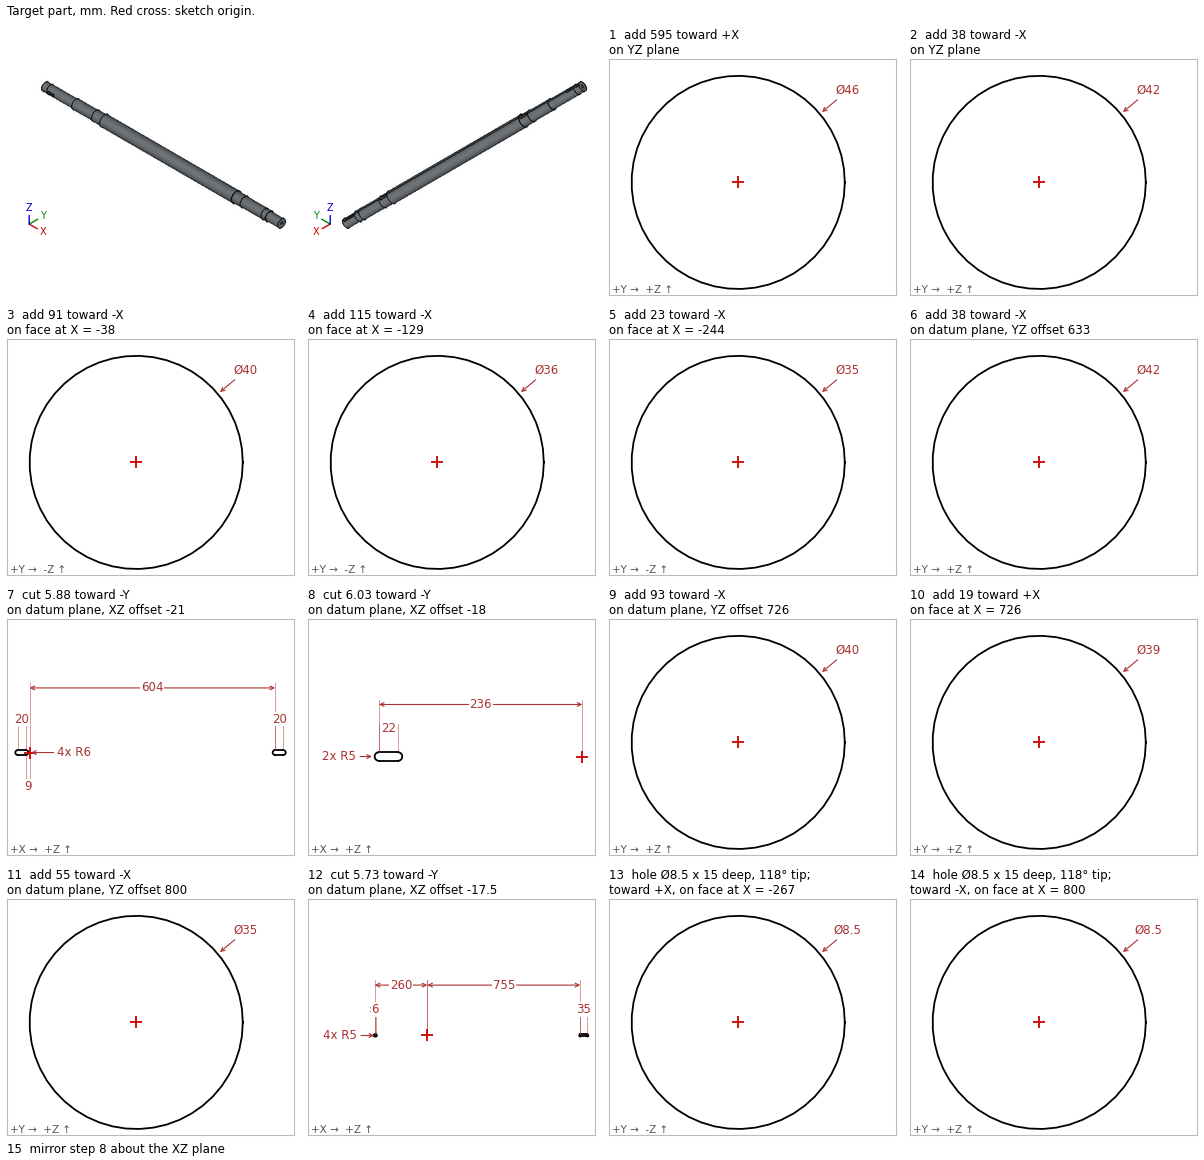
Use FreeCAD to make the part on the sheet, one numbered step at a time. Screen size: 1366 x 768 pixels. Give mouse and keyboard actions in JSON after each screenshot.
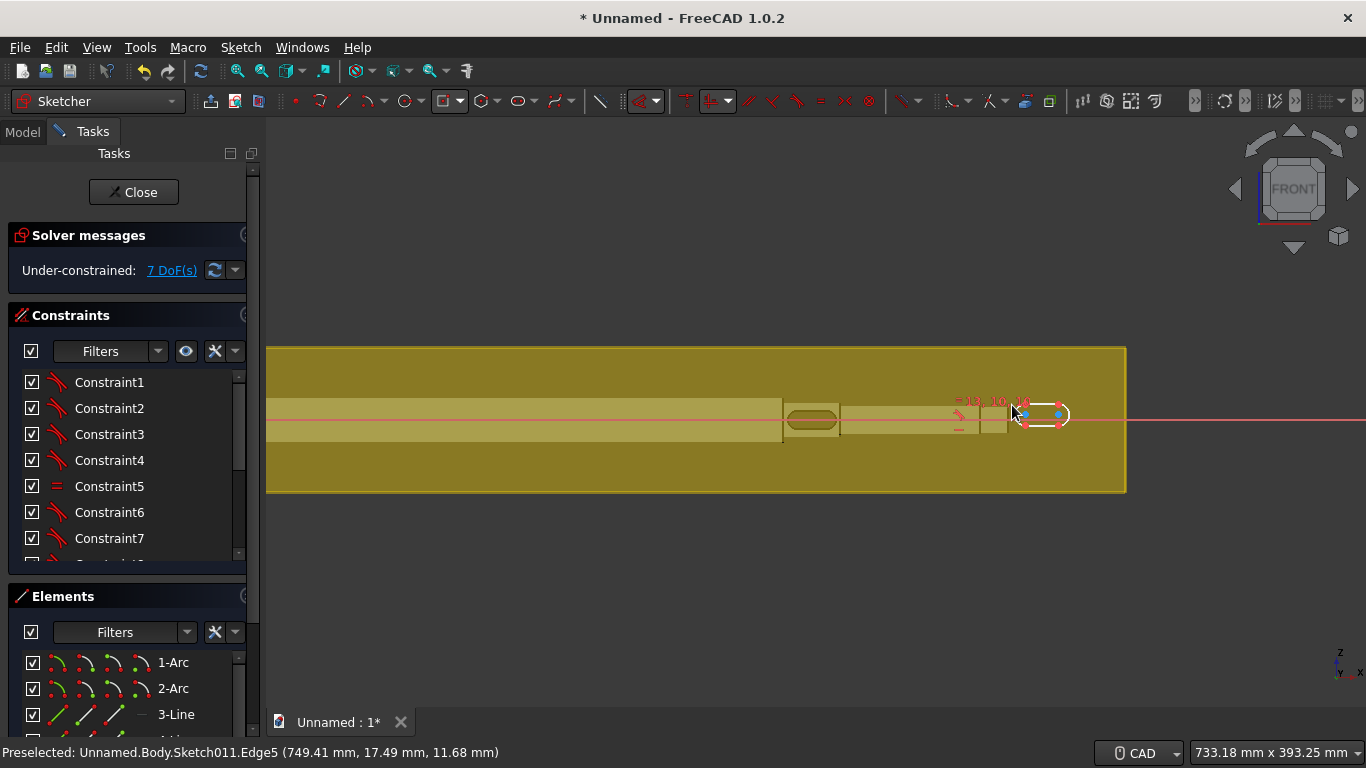
{"action": "scroll", "coordinate": [1015, 407], "scroll_direction": "down", "scroll_amount": 5}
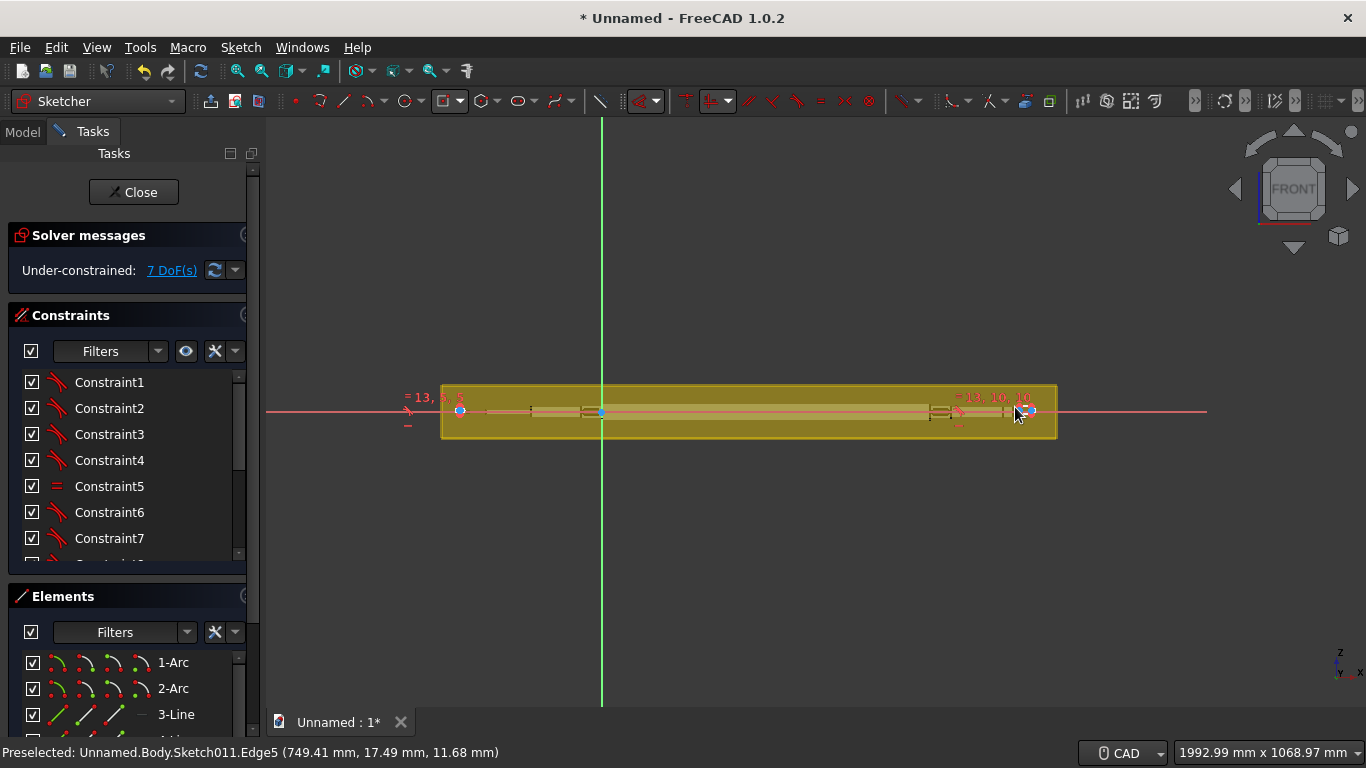
{"action": "scroll", "coordinate": [460, 411], "scroll_direction": "up", "scroll_amount": 14}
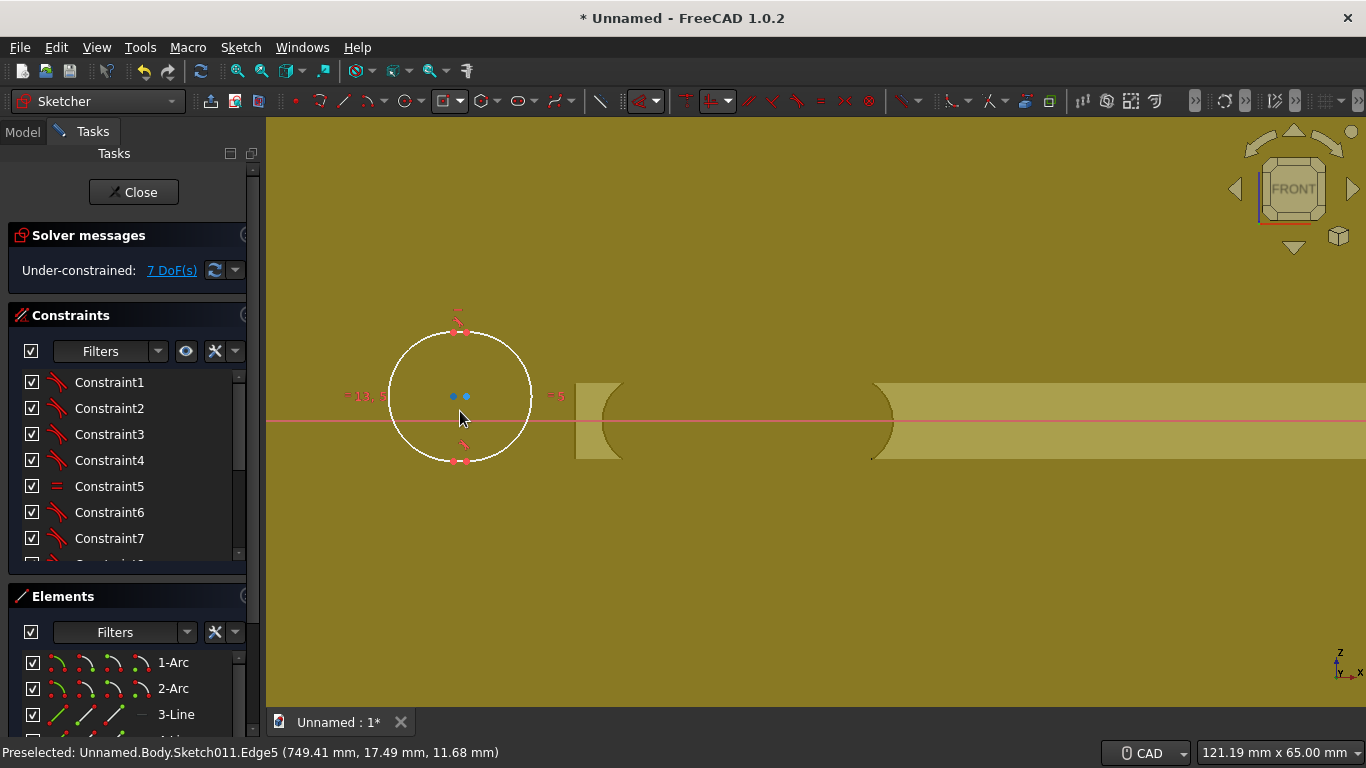
{"action": "left_click", "coordinate": [453, 397]}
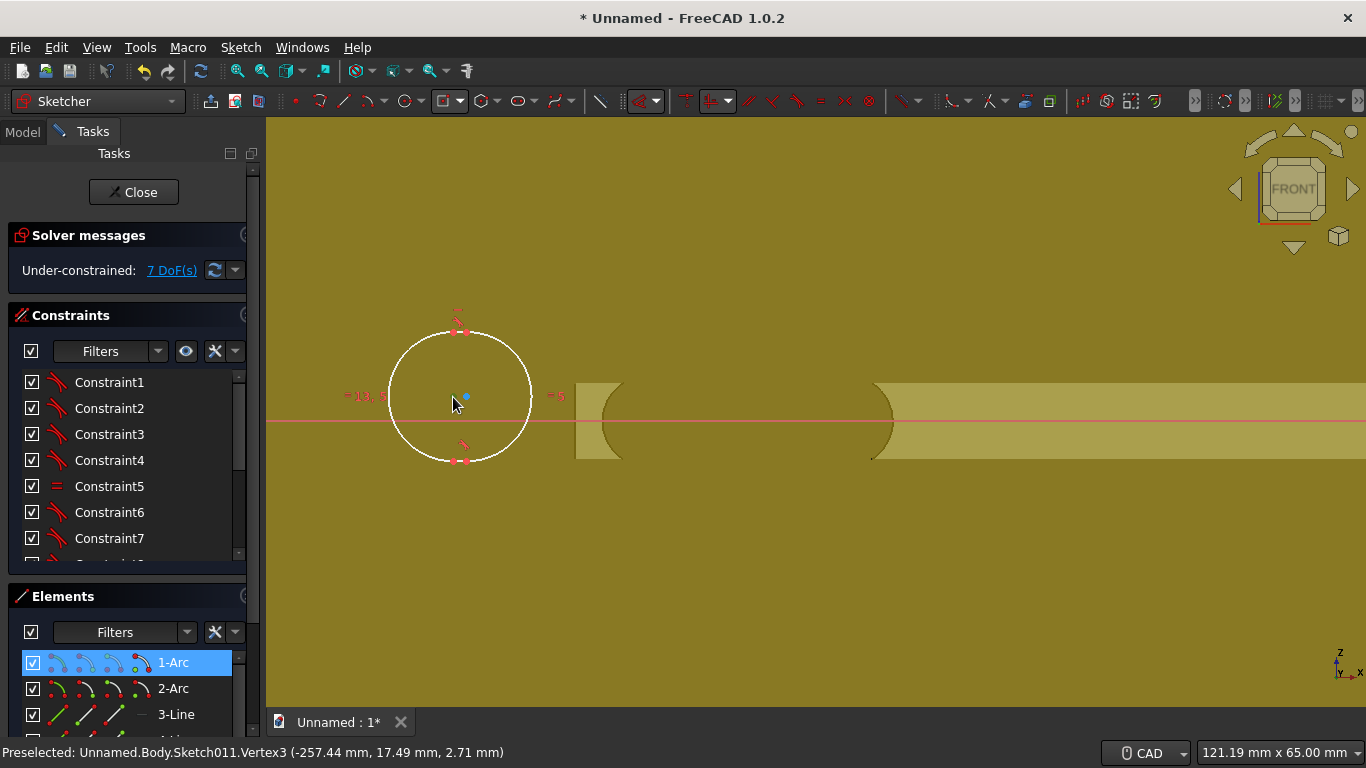
{"action": "left_click", "coordinate": [359, 421]}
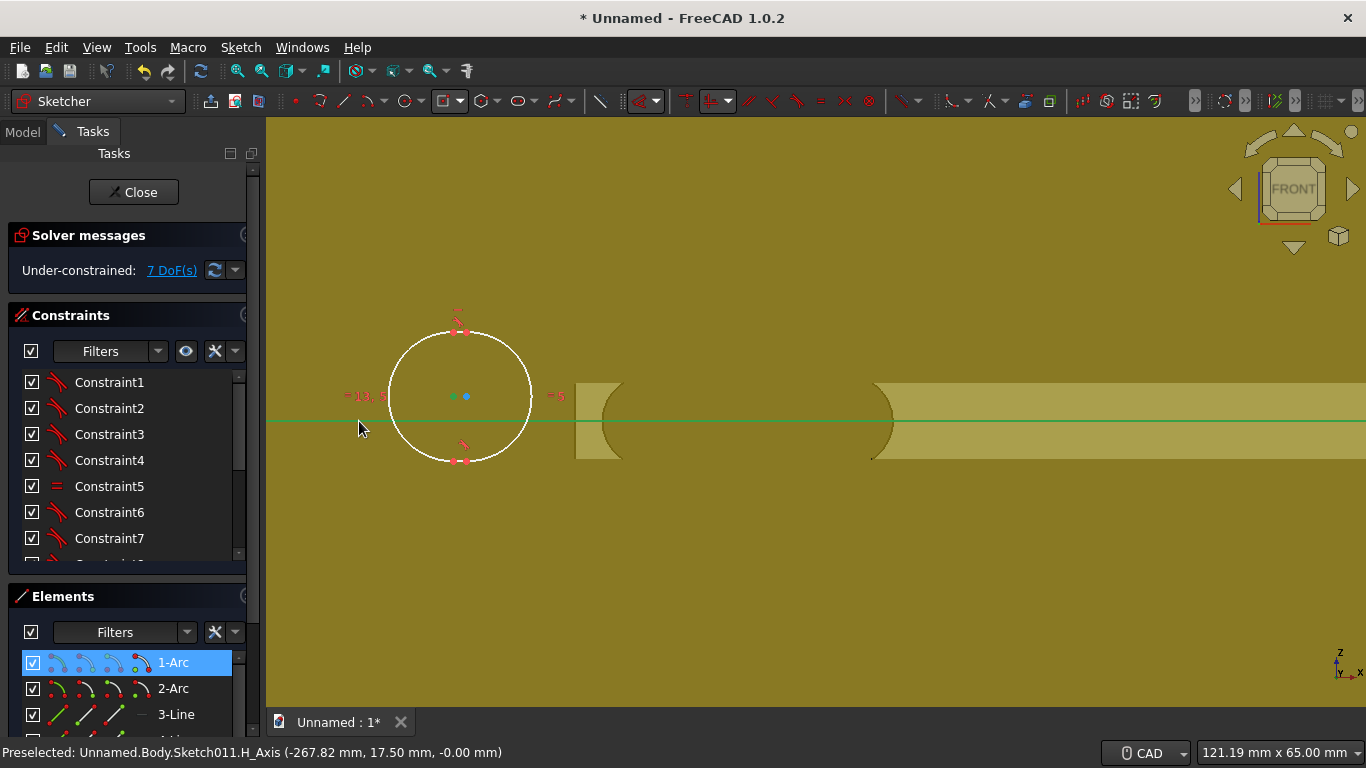
{"action": "key", "text": "c"}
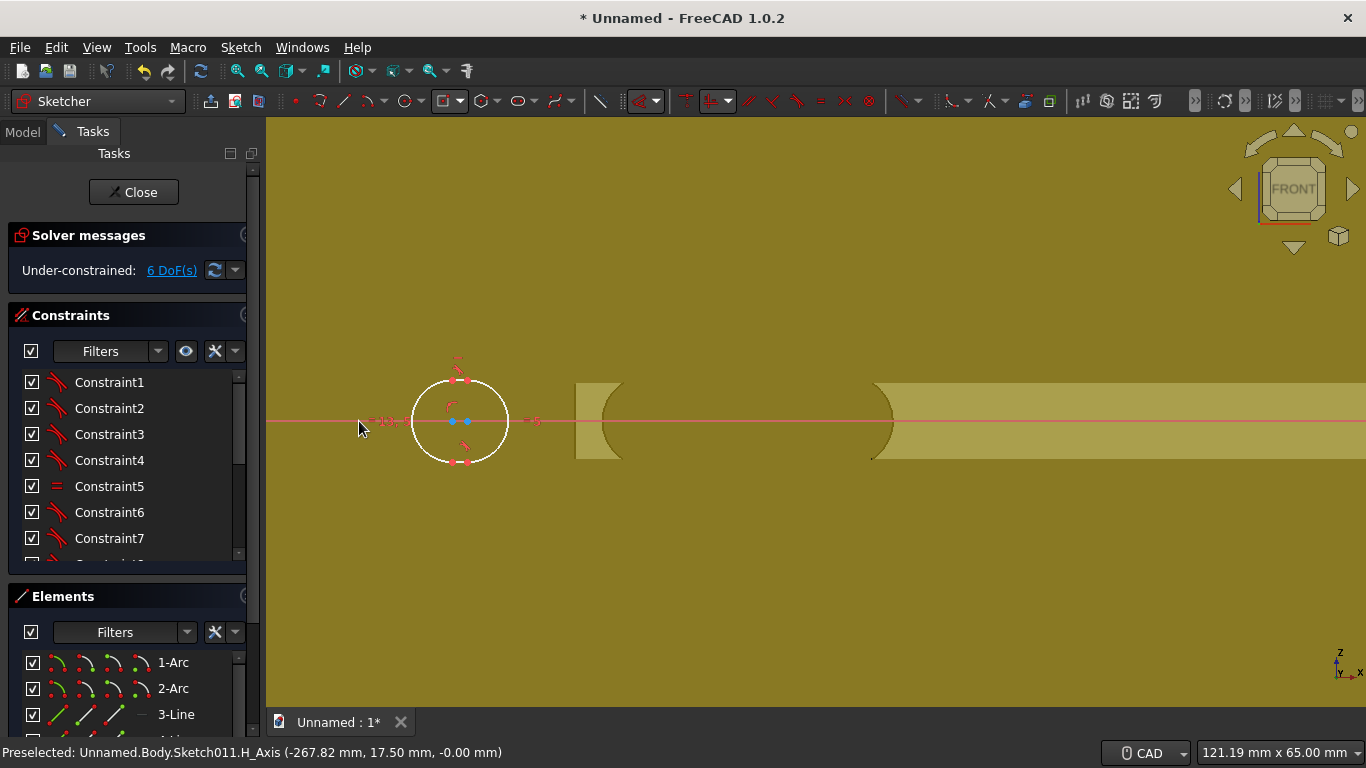
{"action": "scroll", "coordinate": [460, 411], "scroll_direction": "down", "scroll_amount": 14}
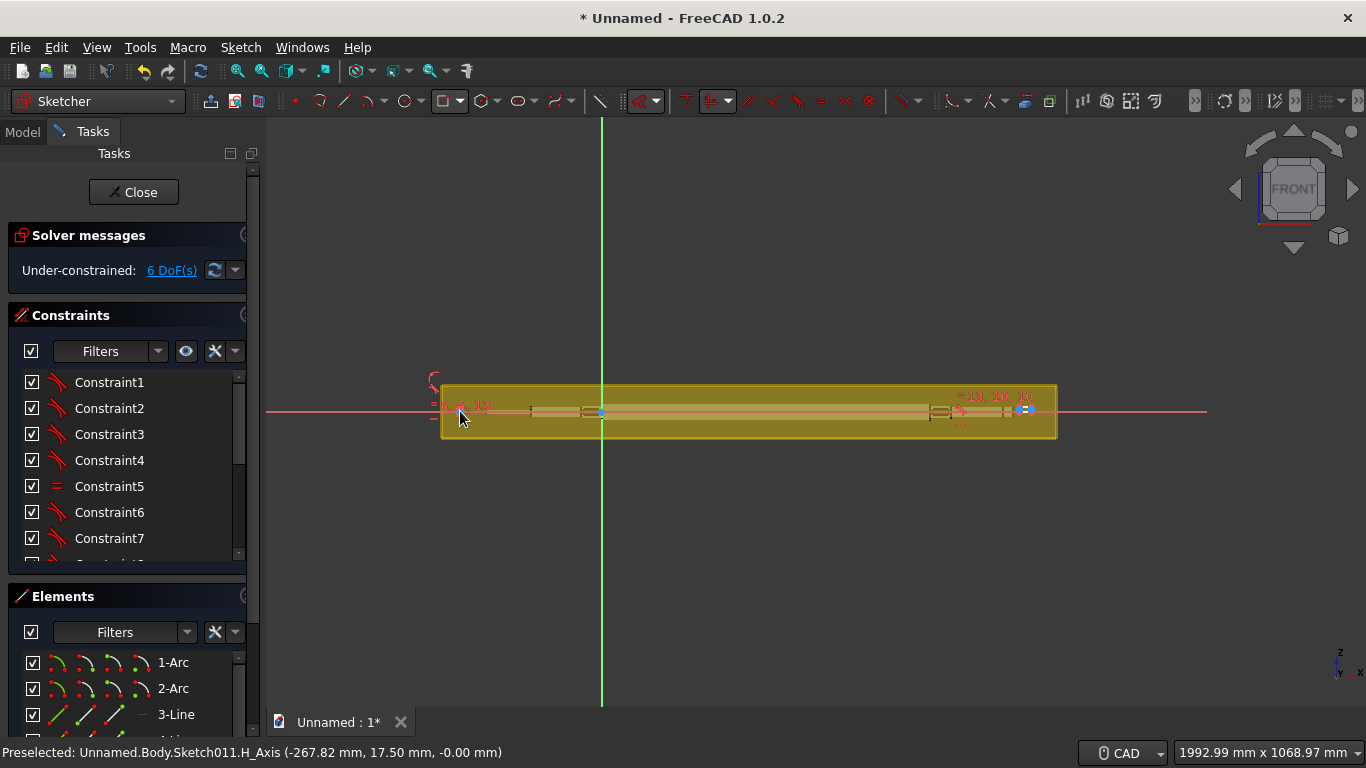
{"action": "scroll", "coordinate": [1019, 410], "scroll_direction": "up", "scroll_amount": 8}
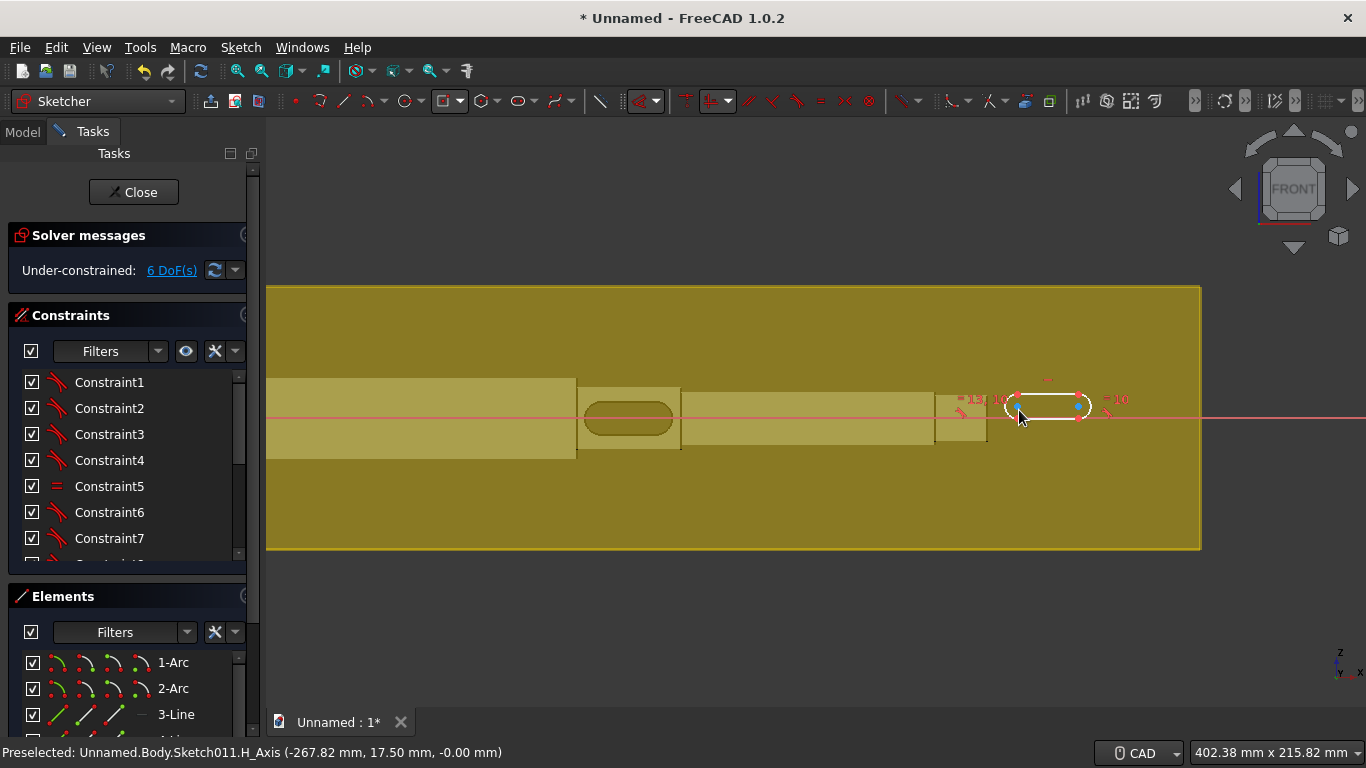
{"action": "left_click", "coordinate": [1018, 406]}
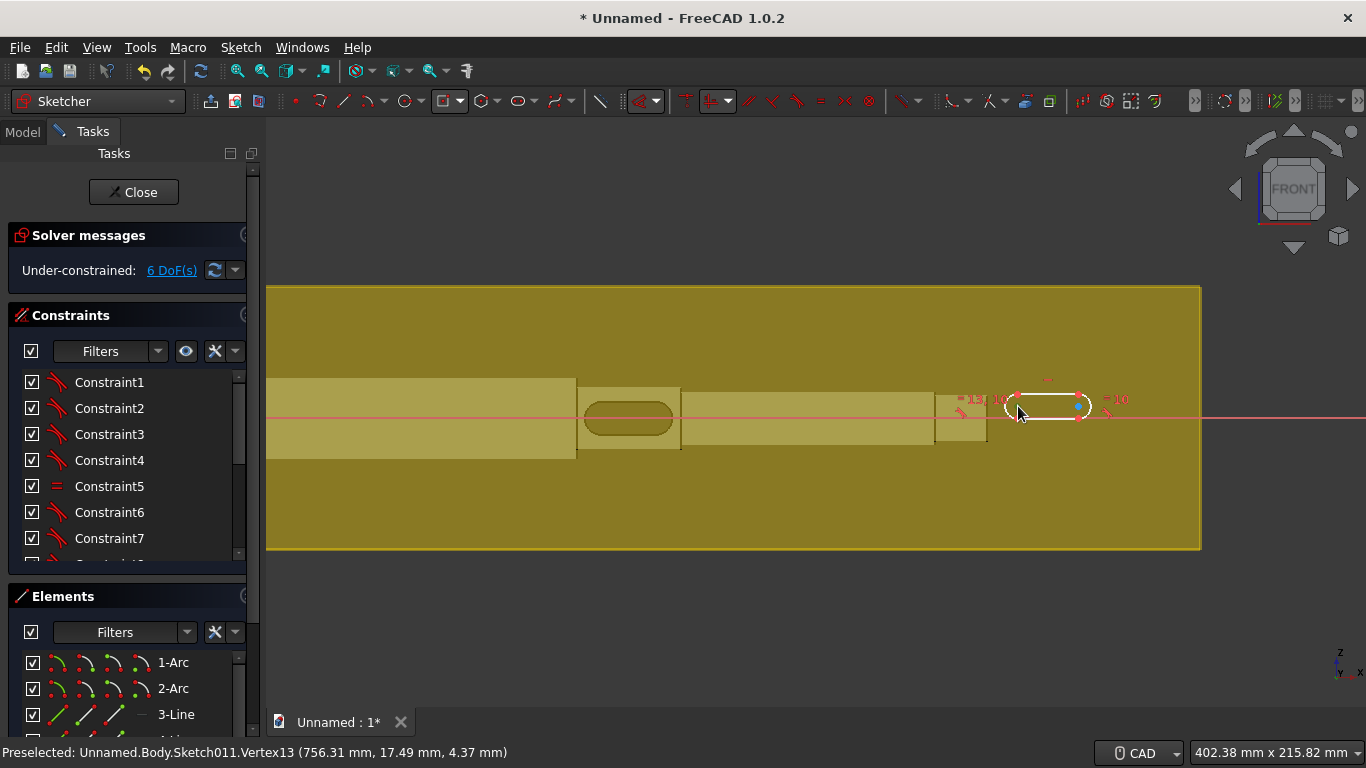
{"action": "left_click", "coordinate": [359, 418]}